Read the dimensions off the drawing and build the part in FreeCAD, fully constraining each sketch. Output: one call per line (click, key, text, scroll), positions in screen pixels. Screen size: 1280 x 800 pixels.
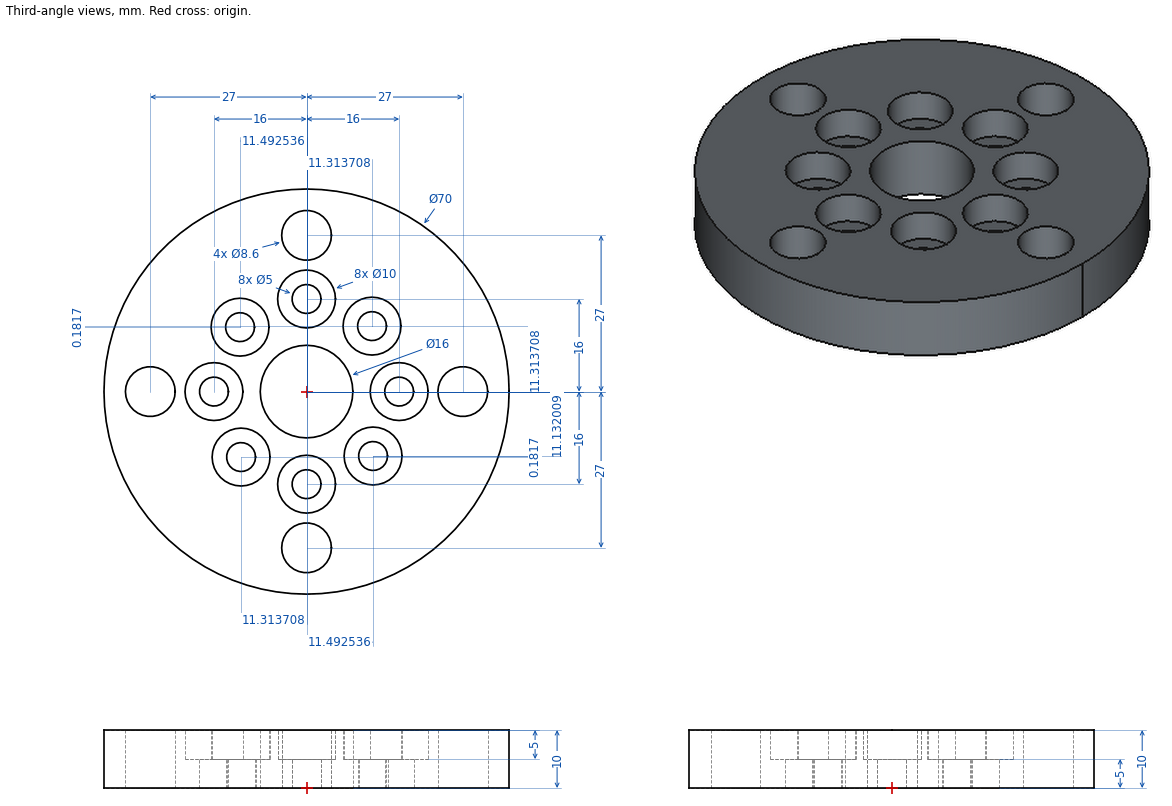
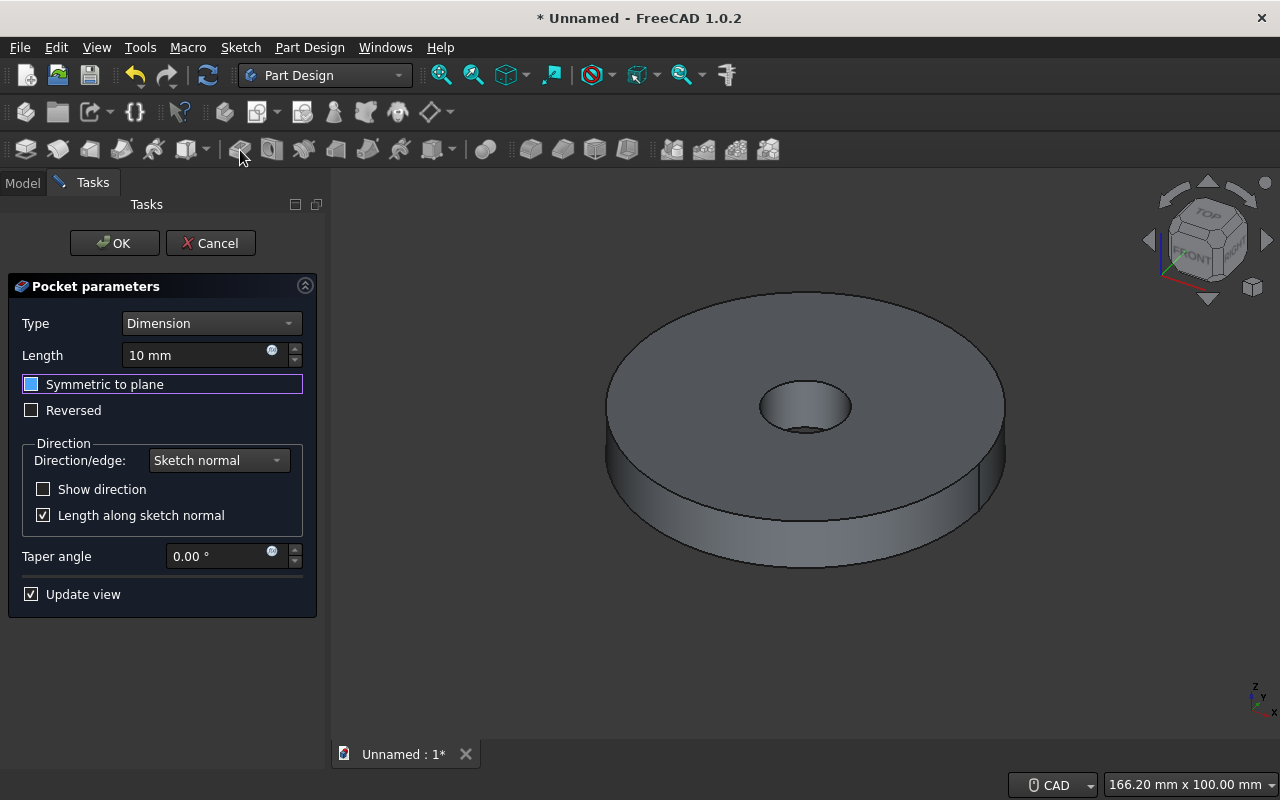
click(115, 243)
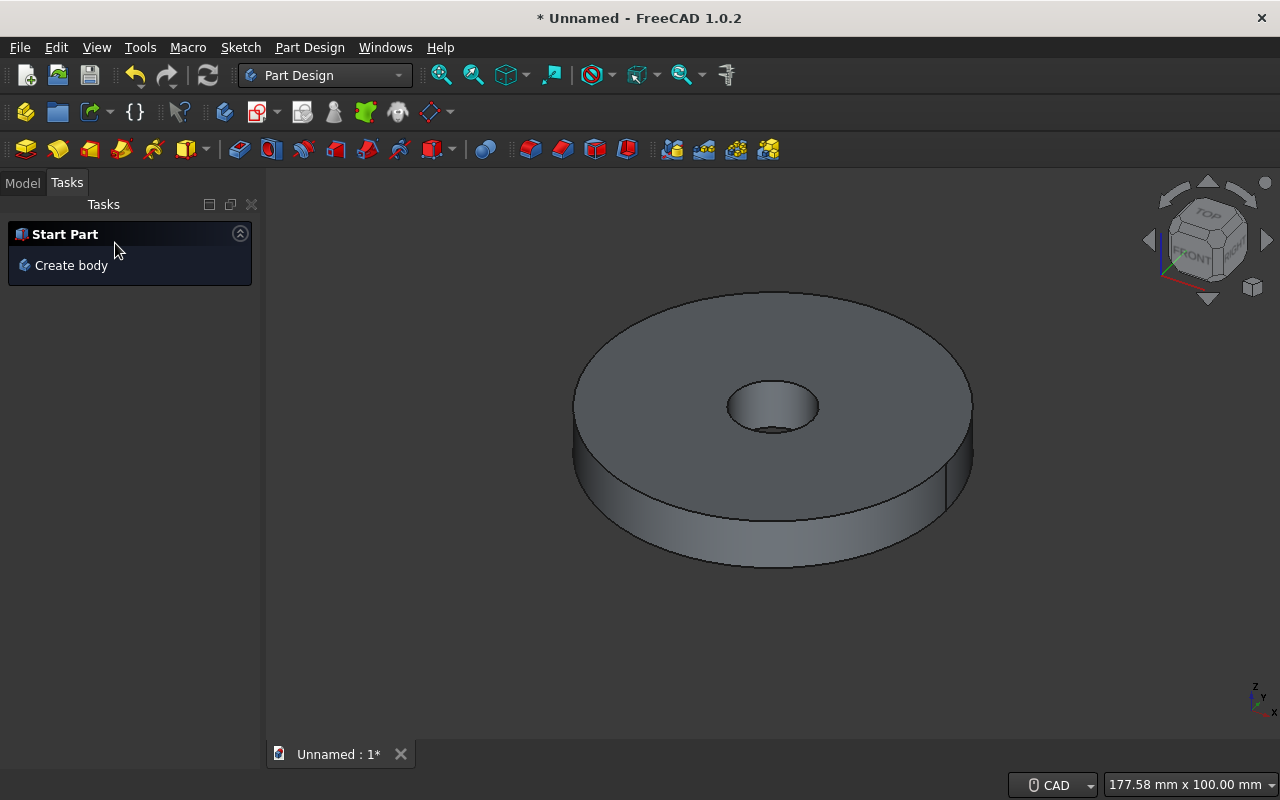
click(765, 479)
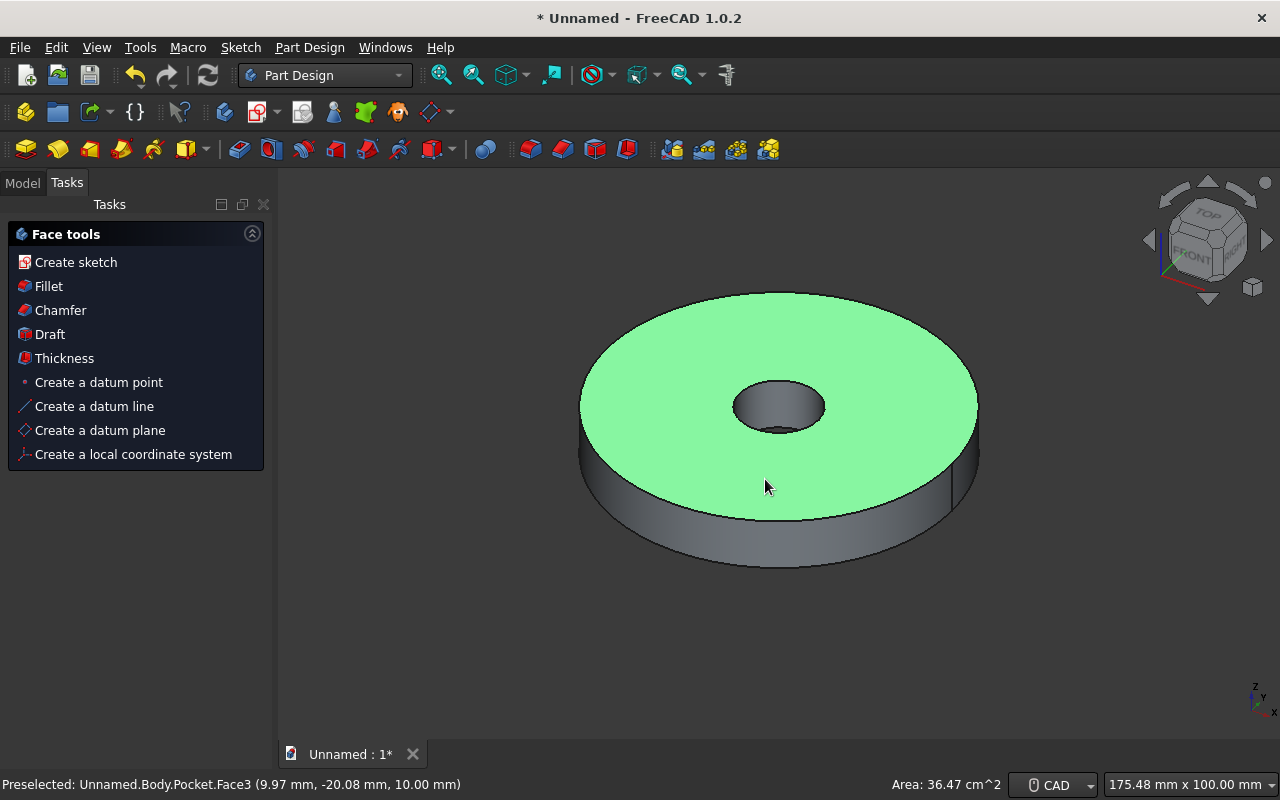
click(258, 112)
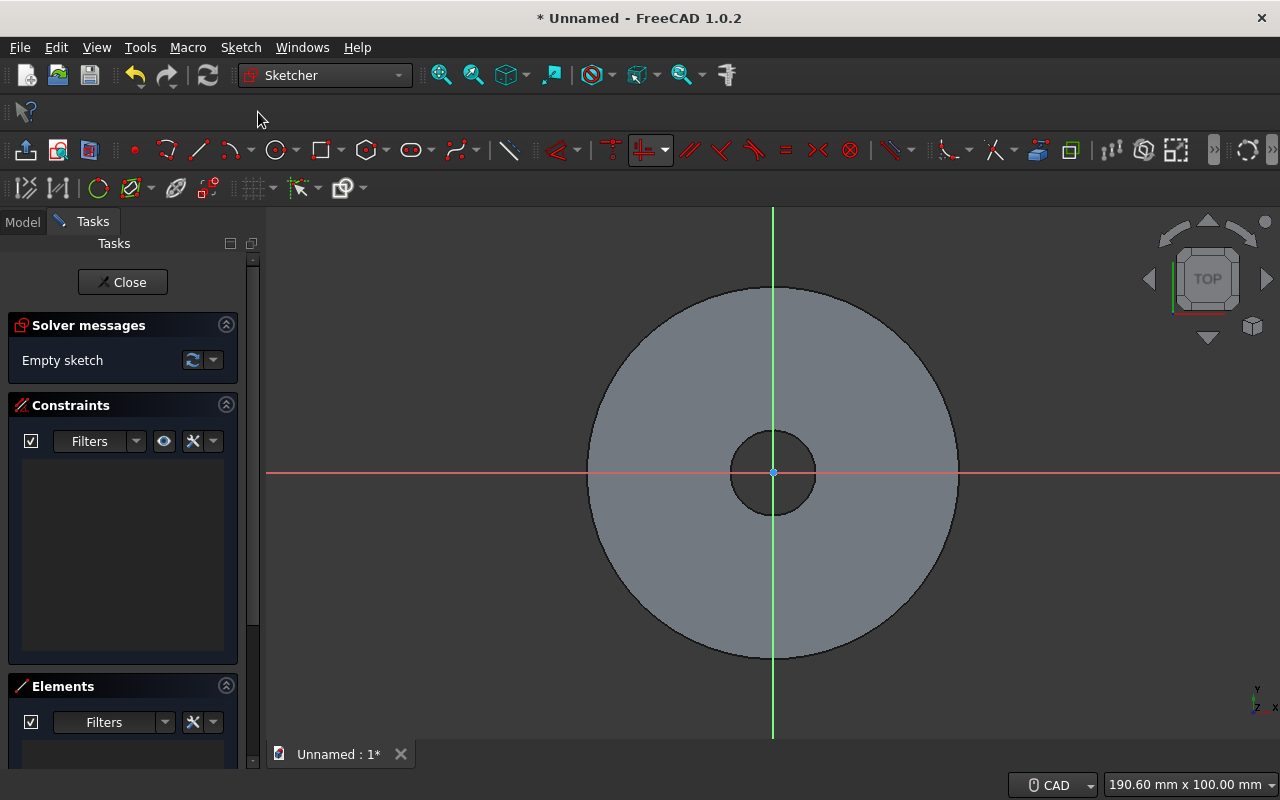
click(276, 150)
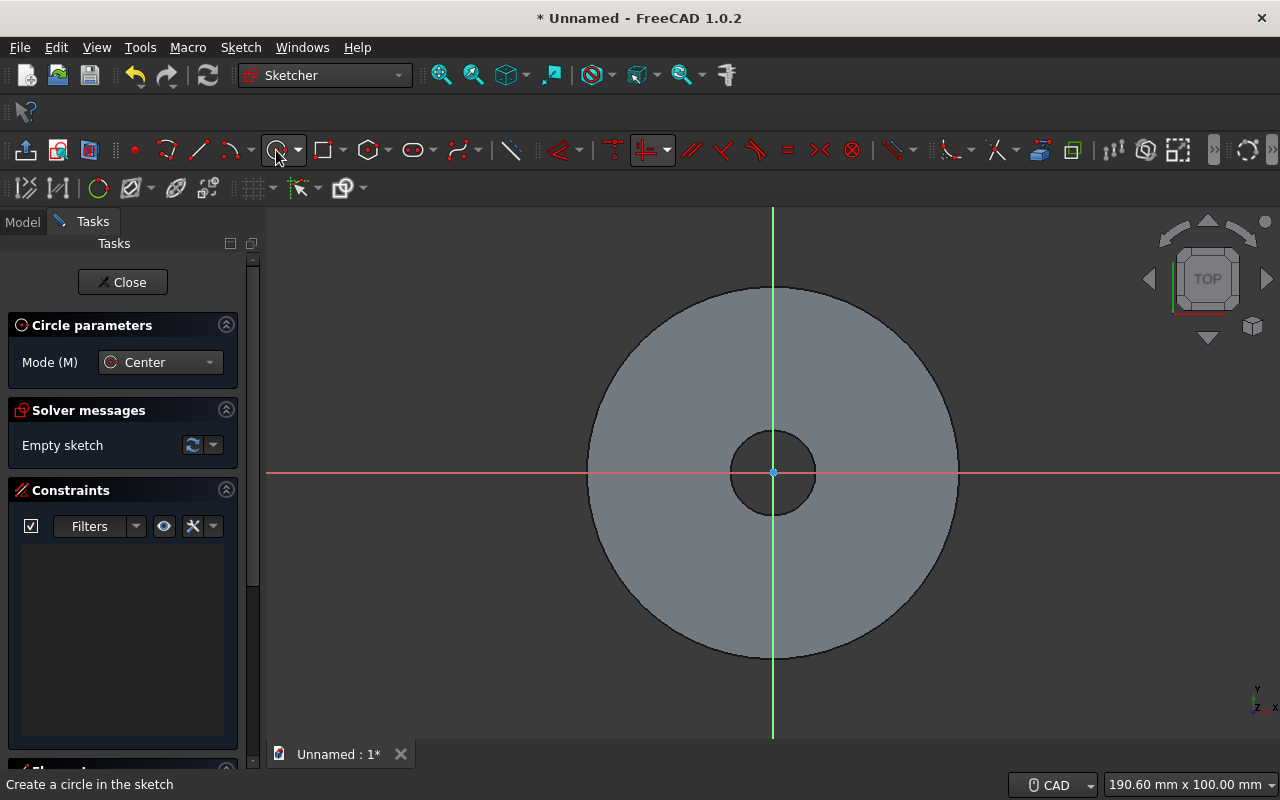
click(773, 329)
move(789, 313)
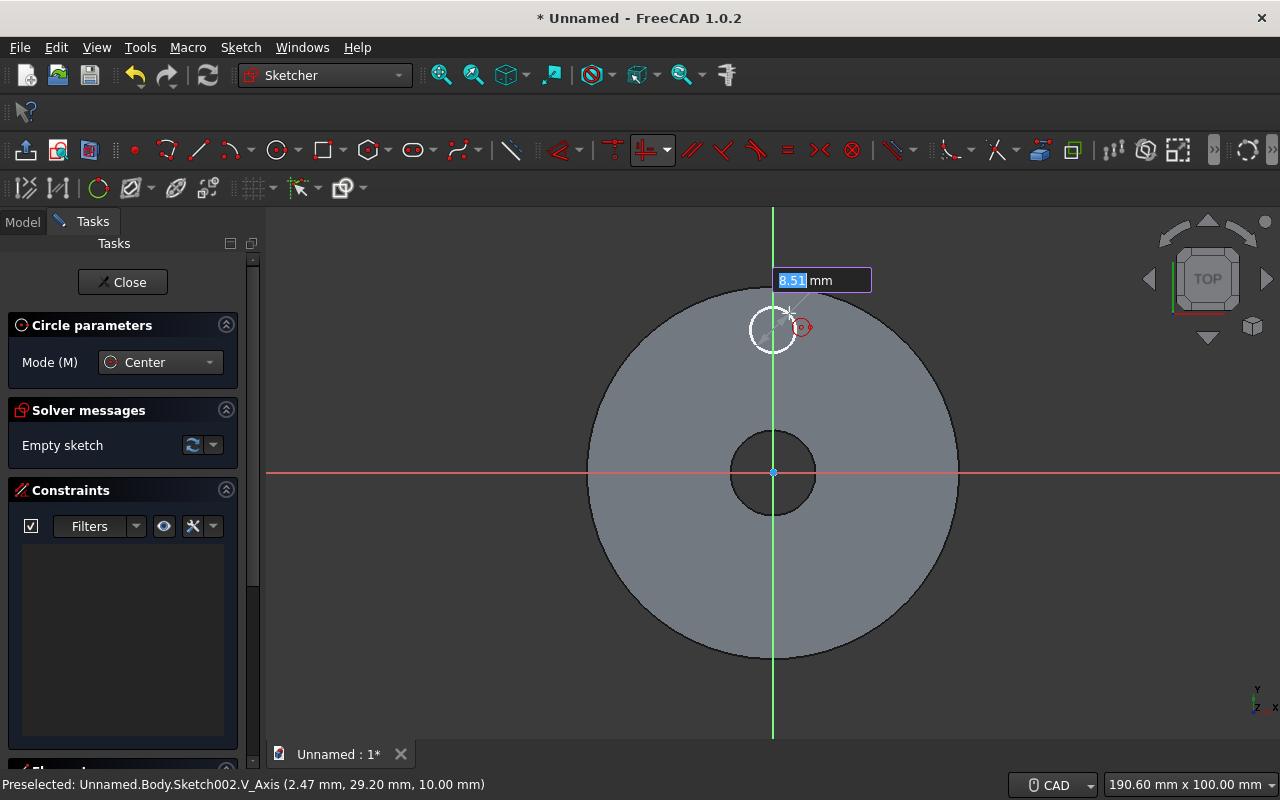
text(8.6)
key(Return)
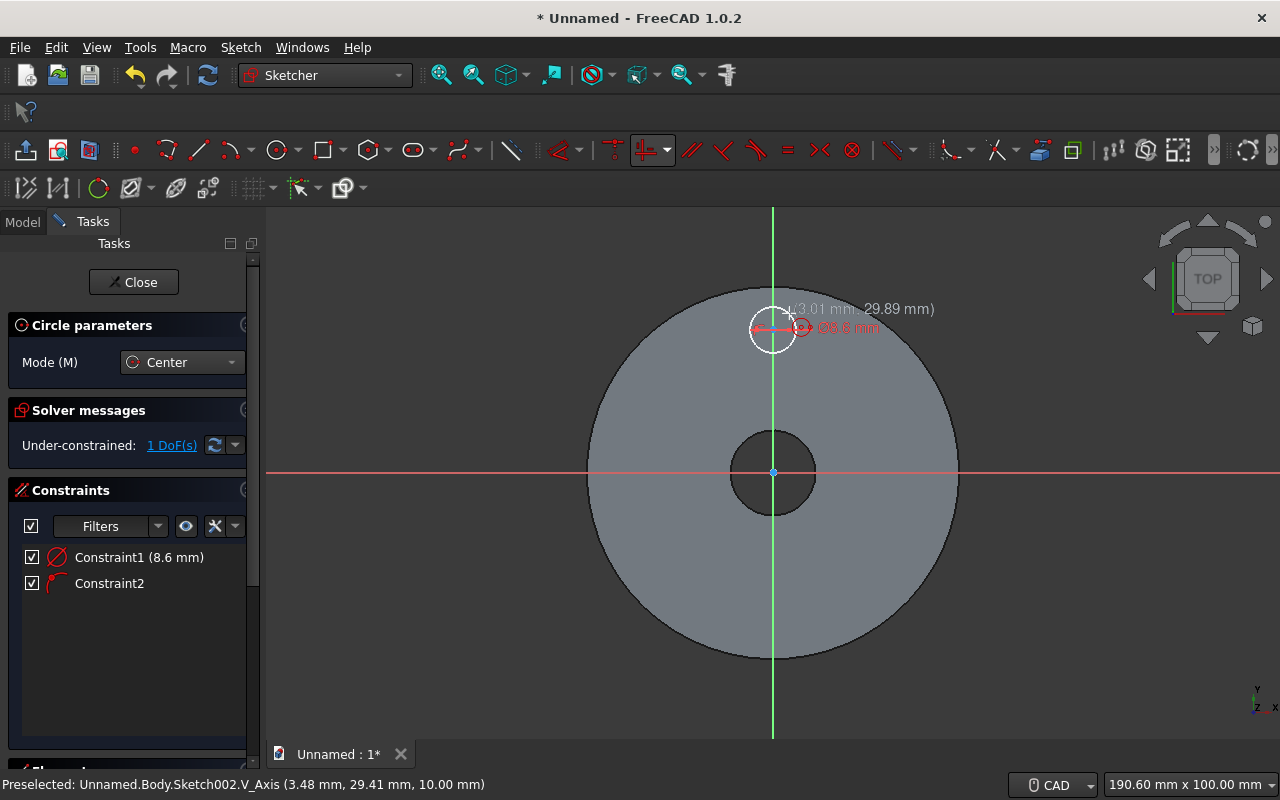
click(917, 473)
move(933, 457)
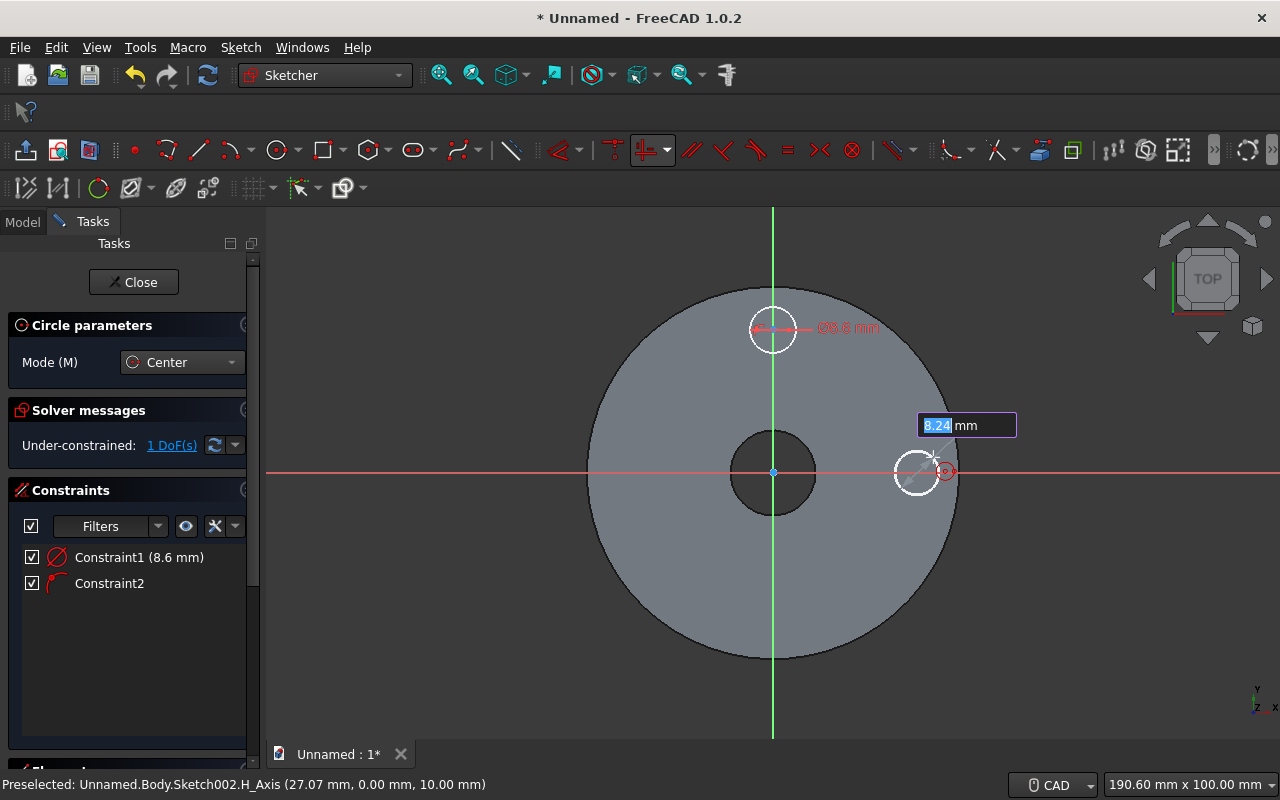
text(8.6)
key(Return)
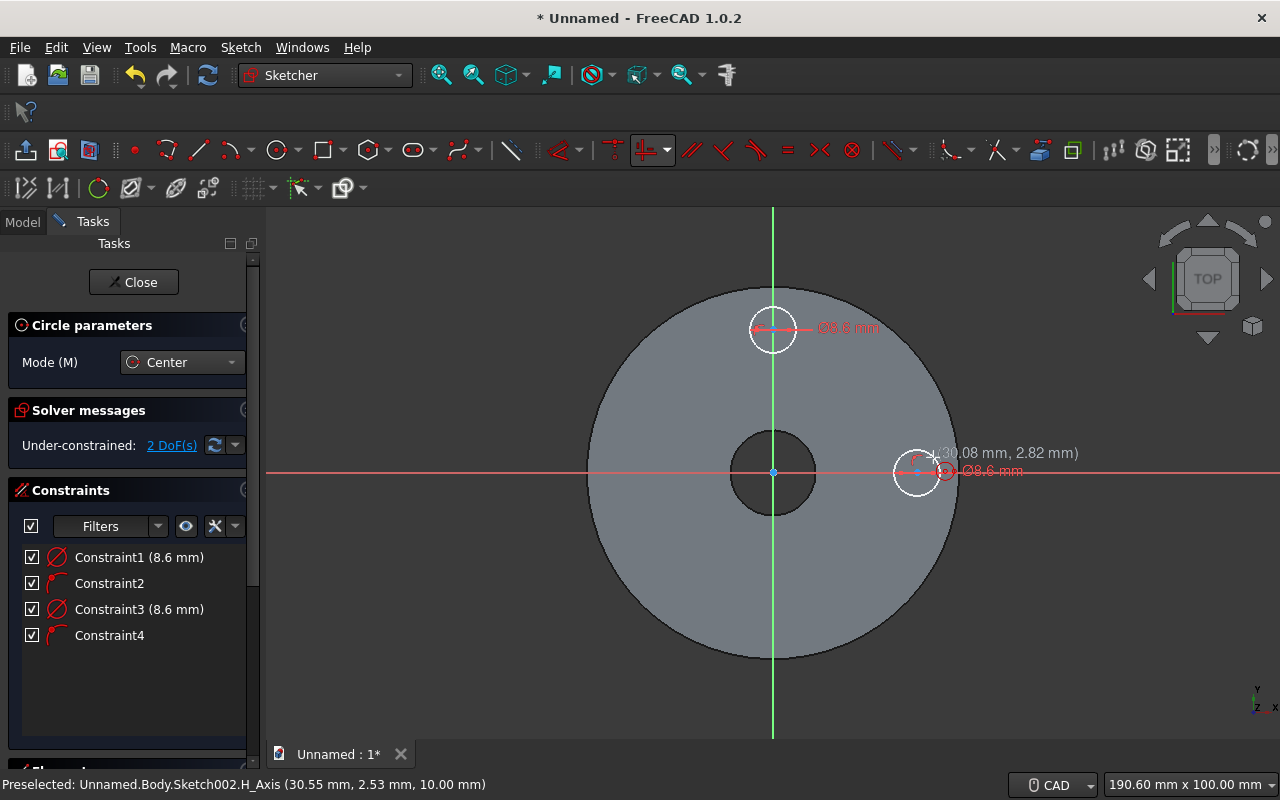
click(773, 617)
move(789, 600)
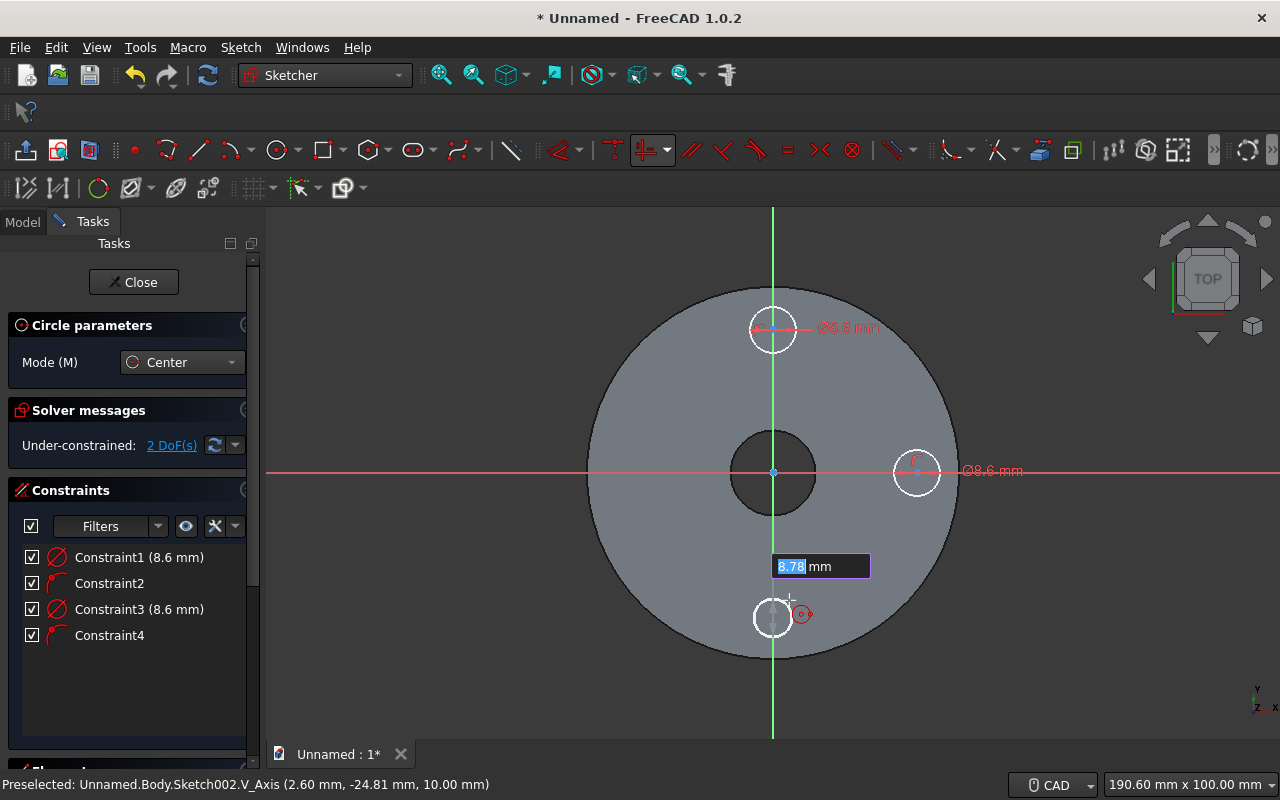
text(8.6)
key(Return)